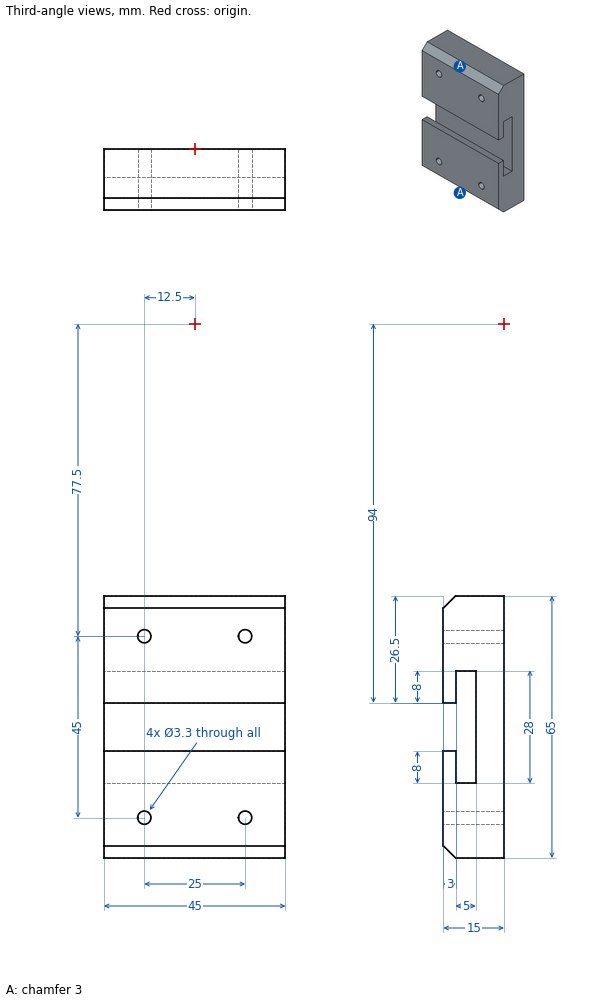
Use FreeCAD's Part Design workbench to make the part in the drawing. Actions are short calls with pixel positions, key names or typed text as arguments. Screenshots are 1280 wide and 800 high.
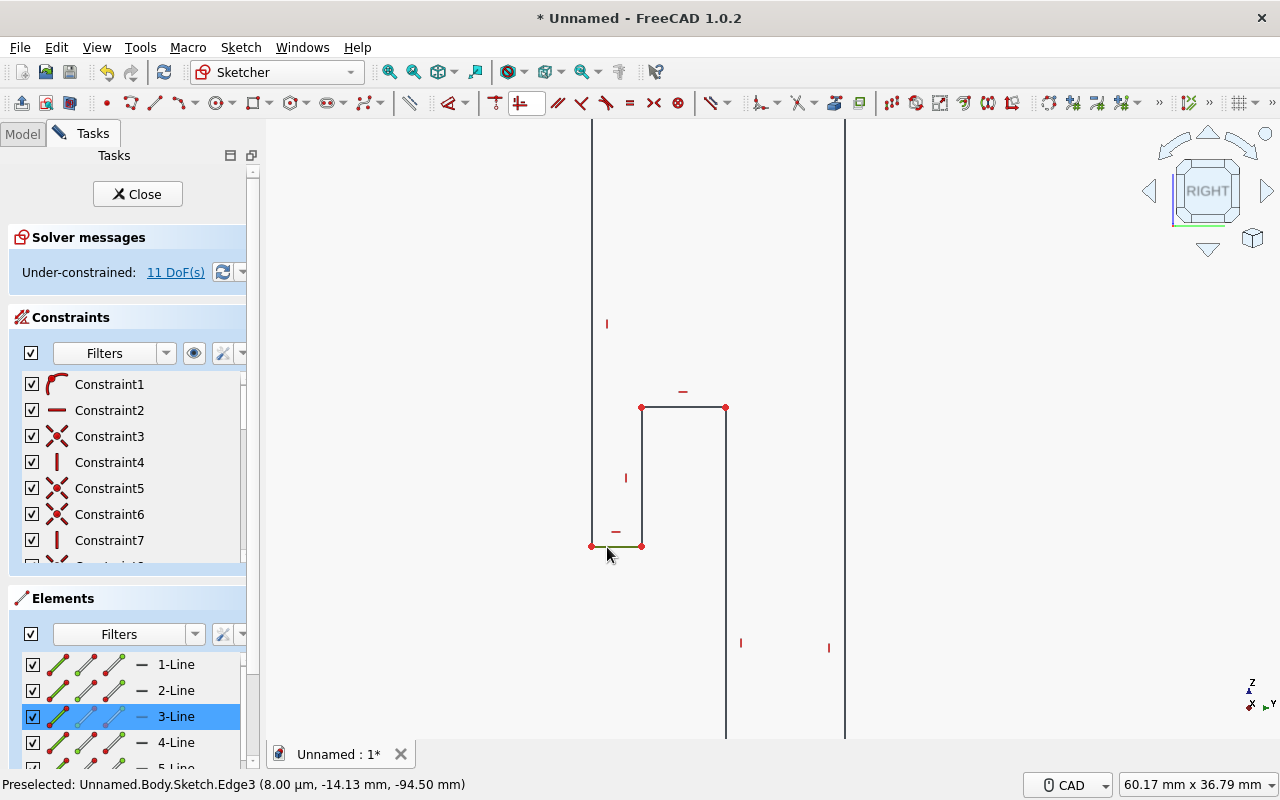
key(l)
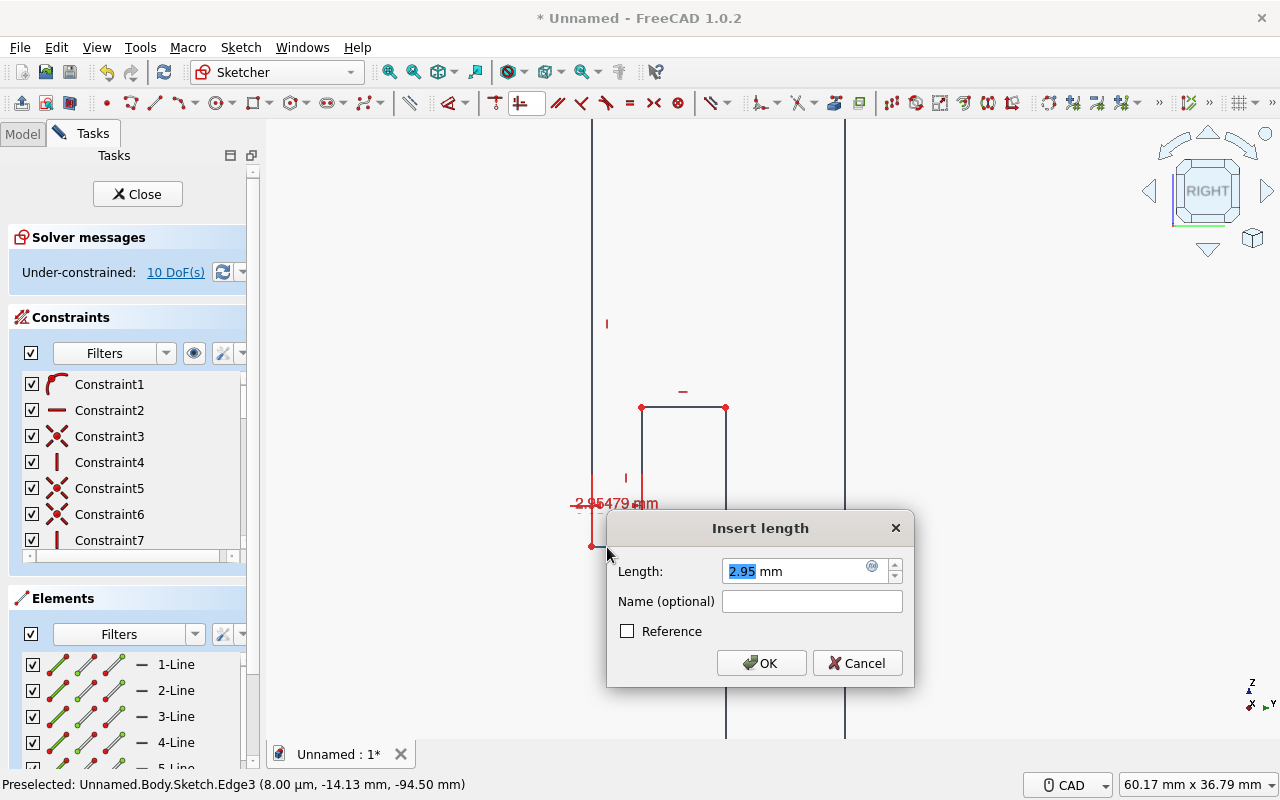
text(3)
key(Return)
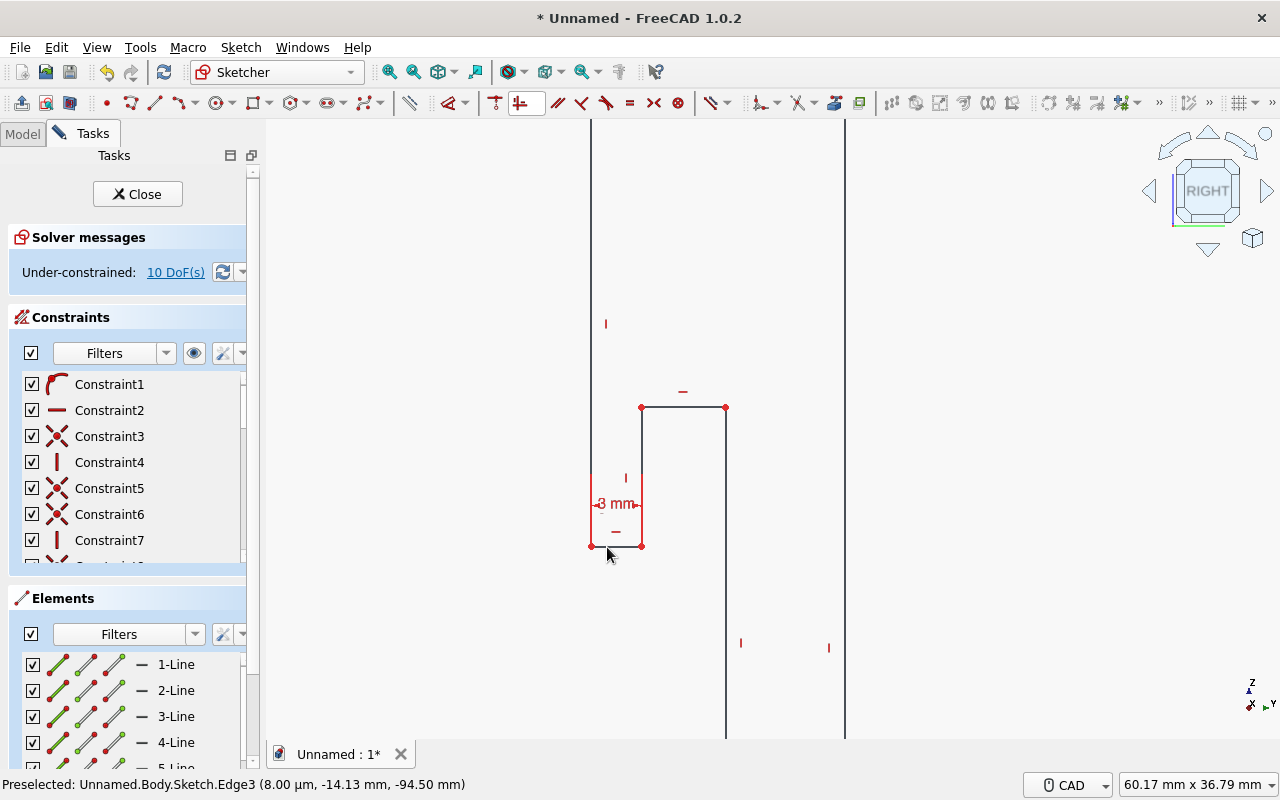
scroll(702, 500, down, 9)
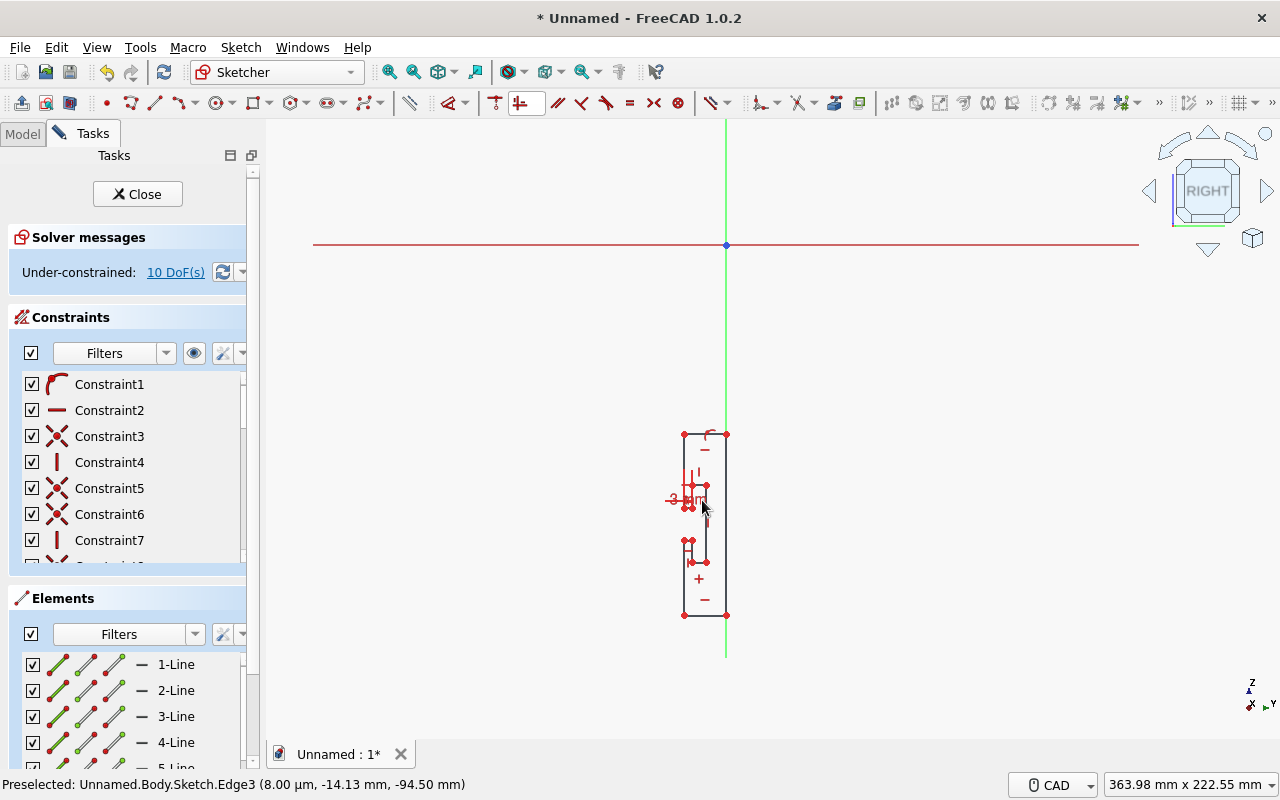
scroll(692, 501, up, 4)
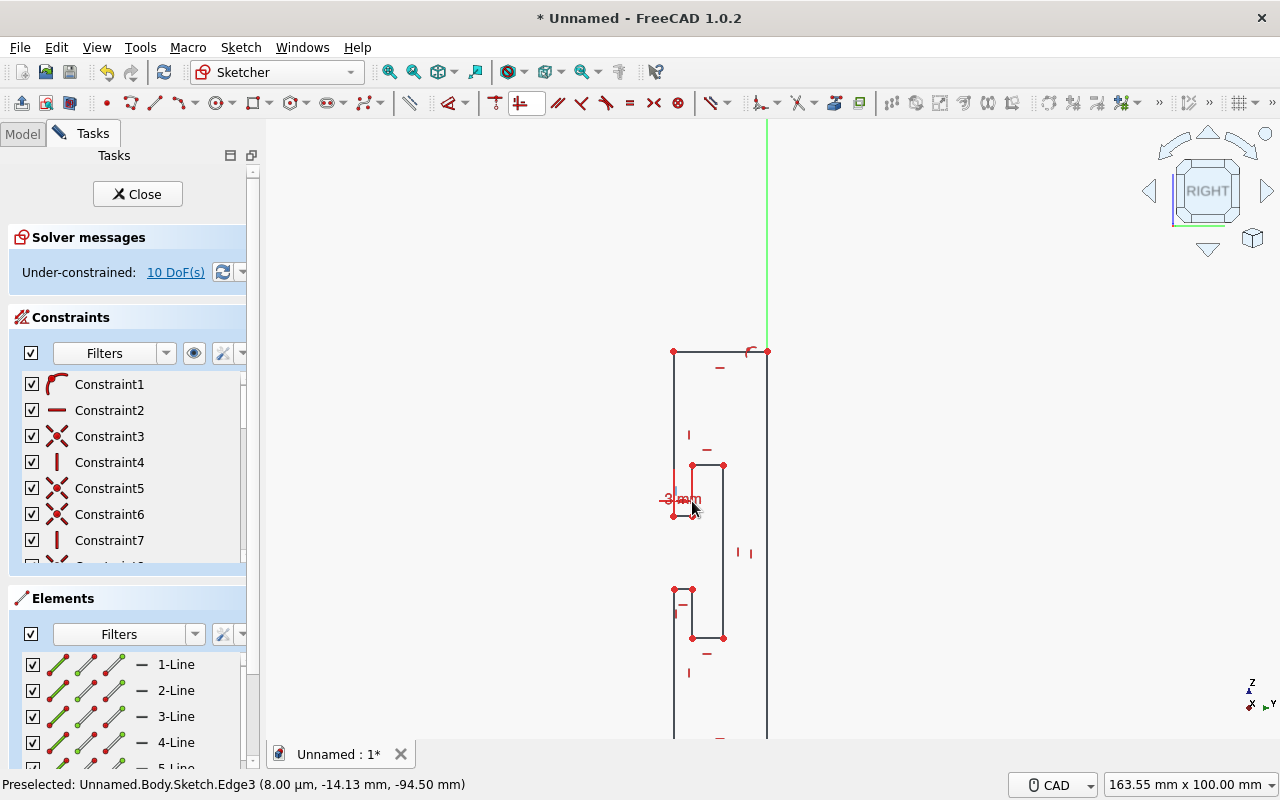
click(692, 480)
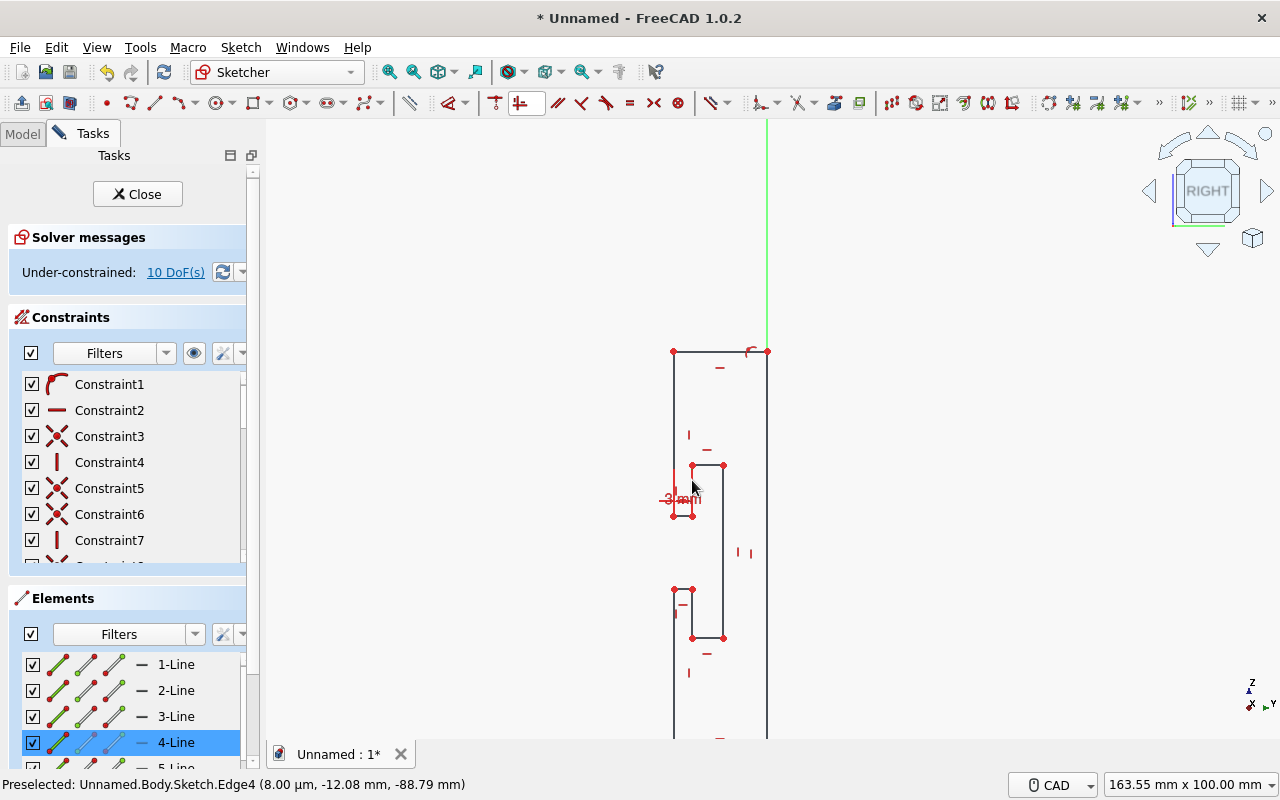
click(468, 104)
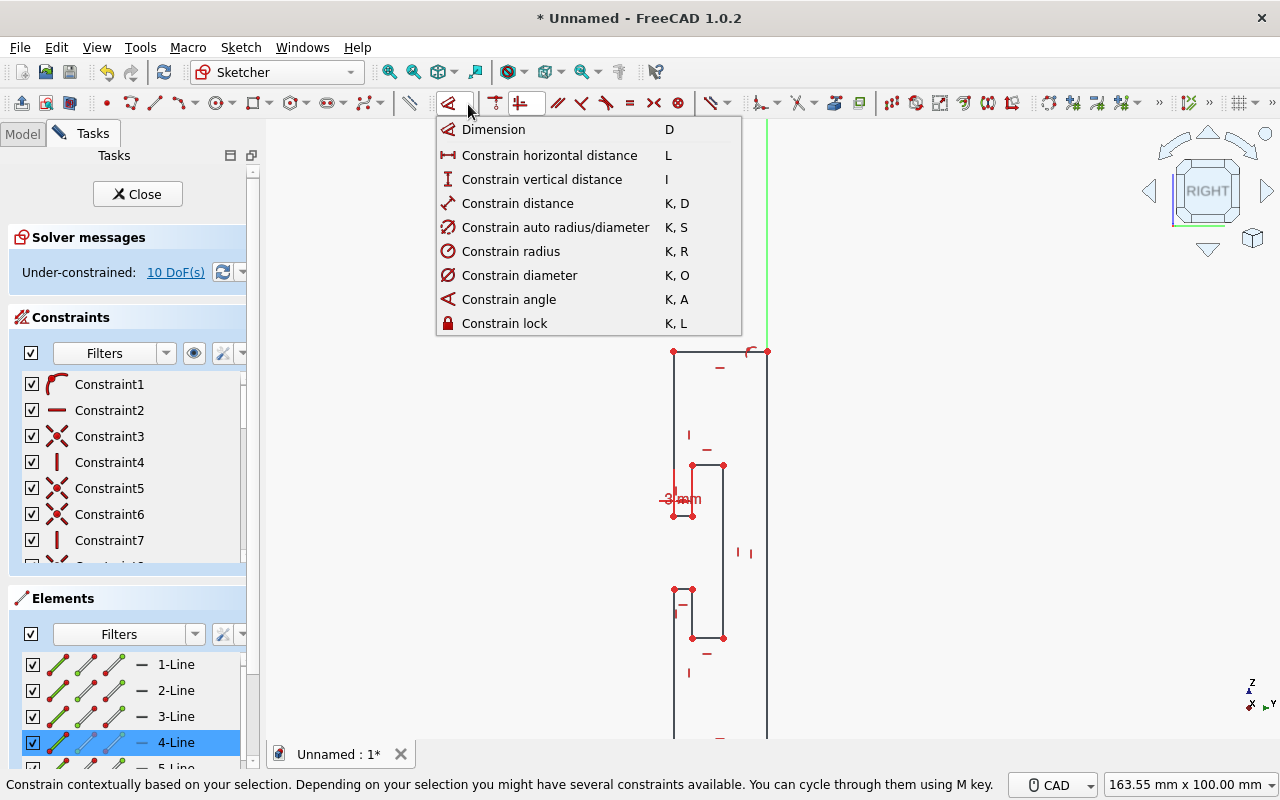
click(589, 179)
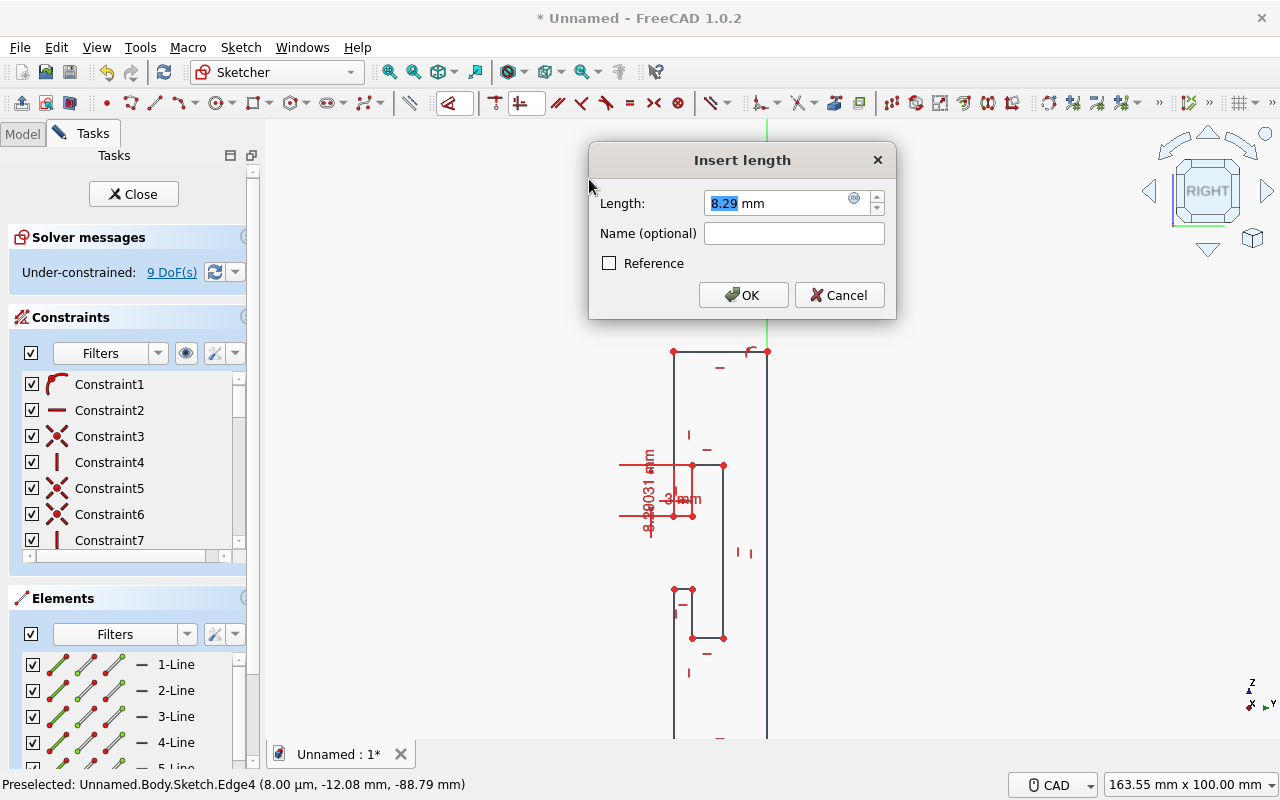
text(8)
key(Return)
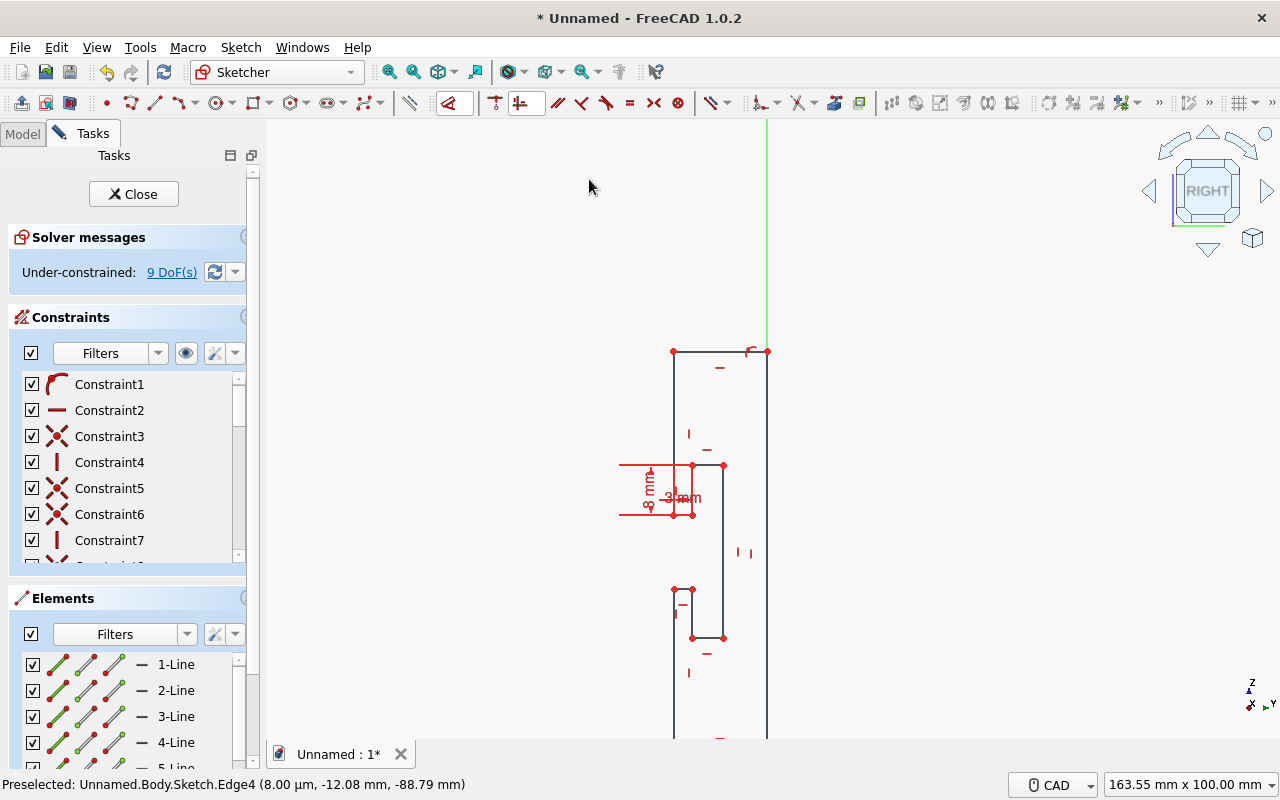
scroll(702, 465, up, 2)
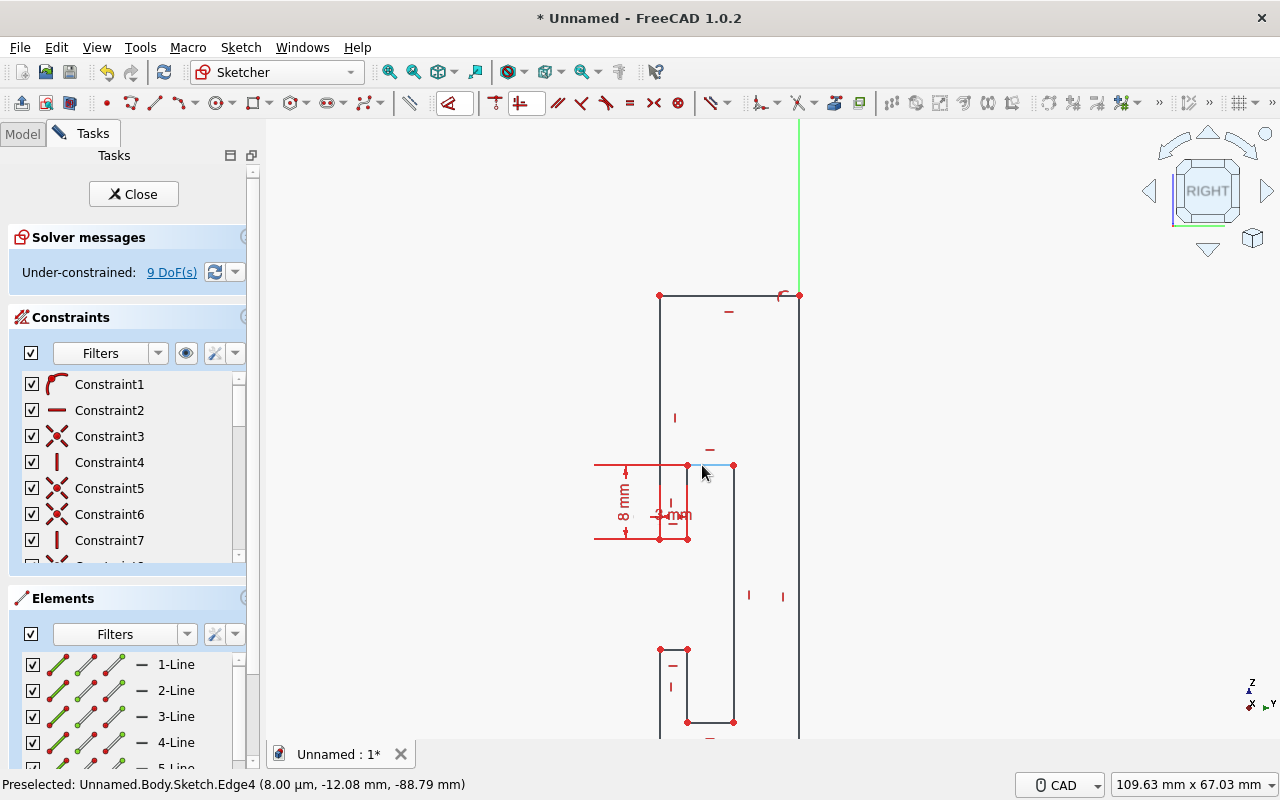
click(701, 465)